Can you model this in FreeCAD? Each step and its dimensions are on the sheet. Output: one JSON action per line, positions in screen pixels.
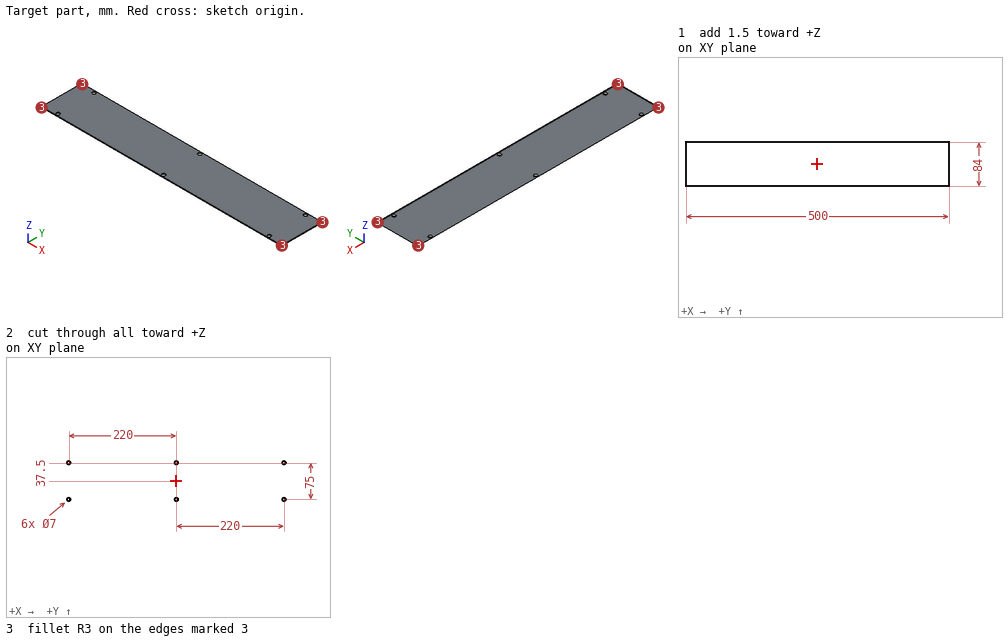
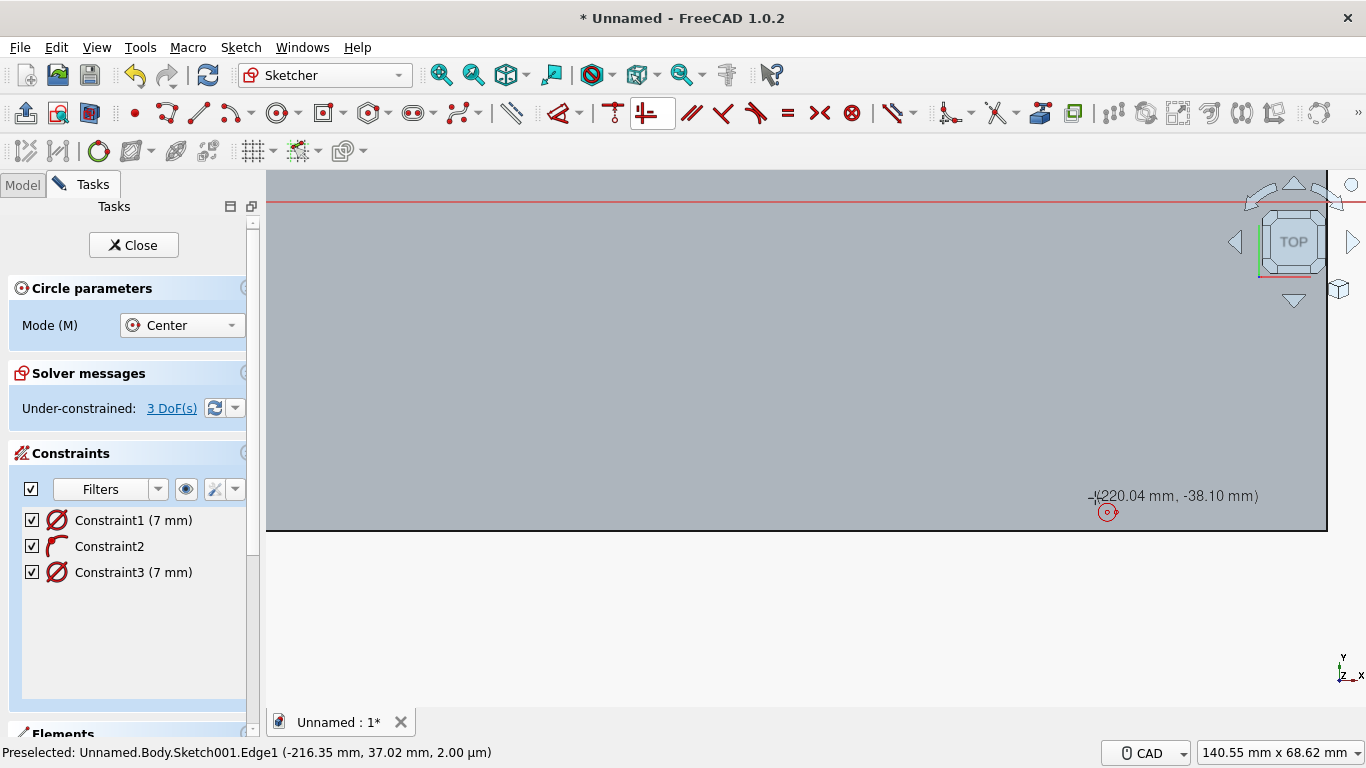
{"action": "scroll", "coordinate": [1096, 498], "scroll_direction": "down", "scroll_amount": 8}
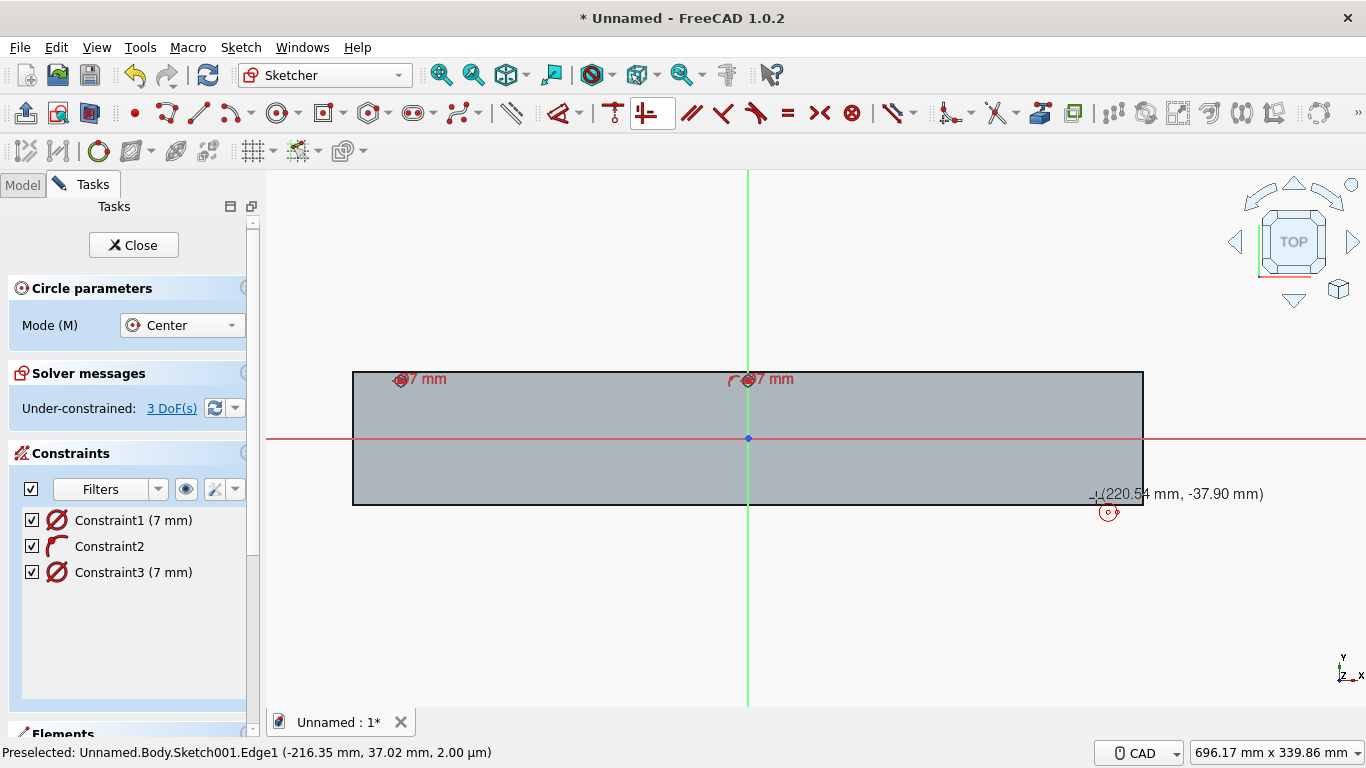
{"action": "left_click", "coordinate": [1096, 498]}
{"action": "mouse_move", "coordinate": [1100, 494]}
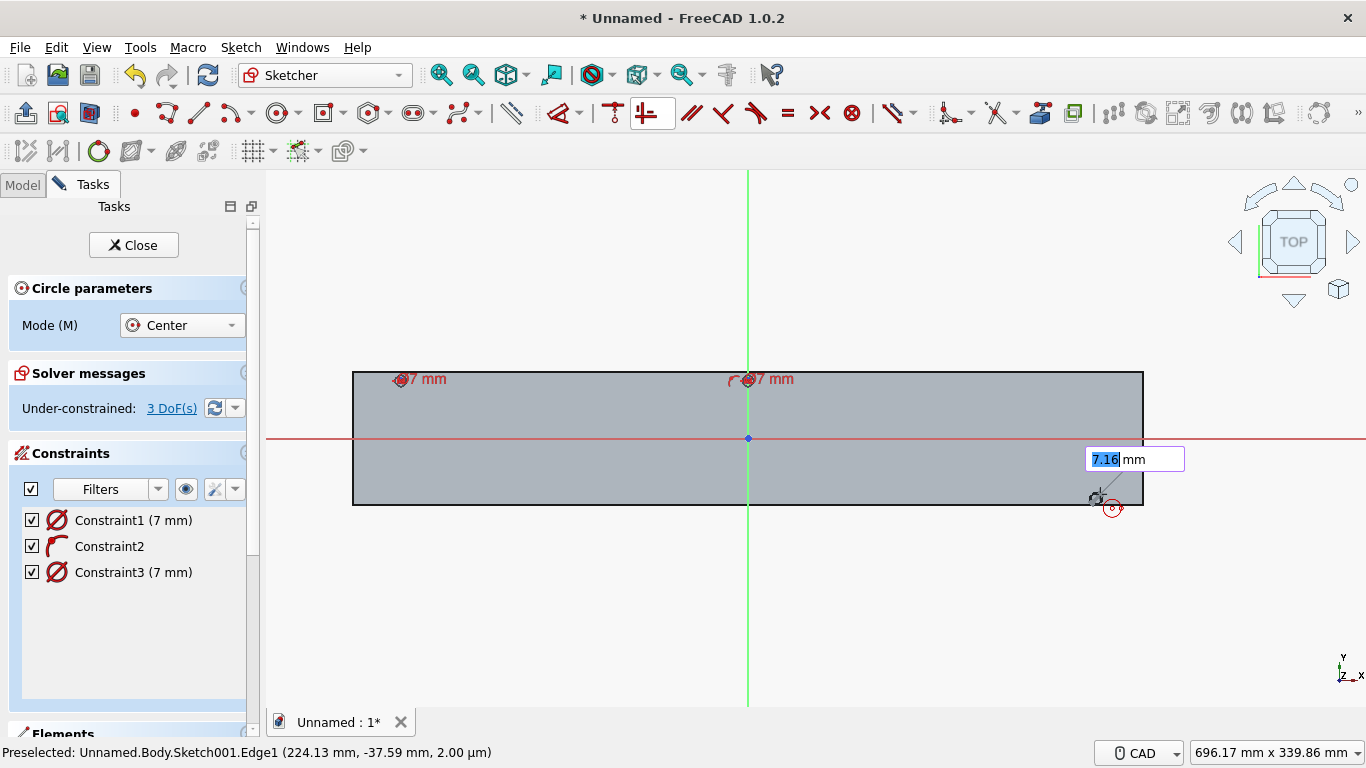
{"action": "type", "text": "7"}
{"action": "key", "text": "Return"}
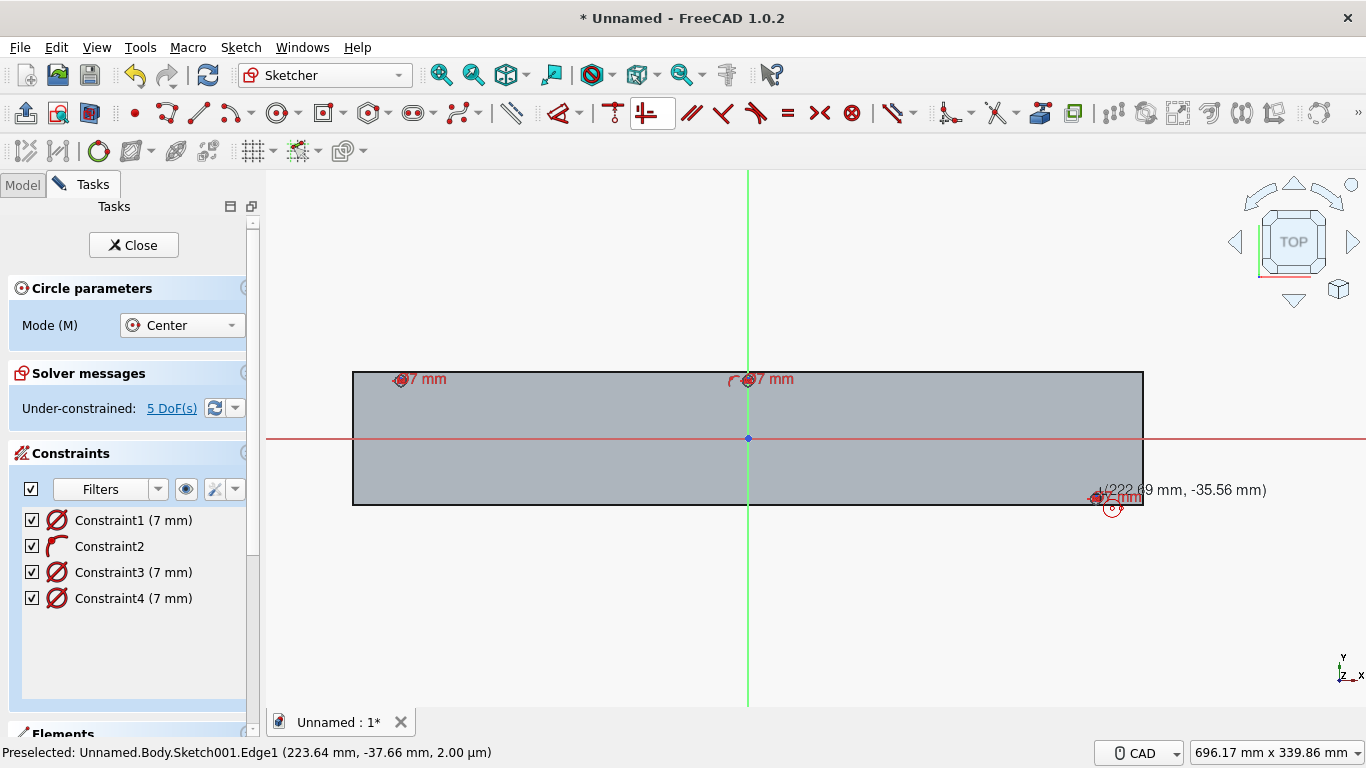
{"action": "scroll", "coordinate": [401, 498], "scroll_direction": "up", "scroll_amount": 8}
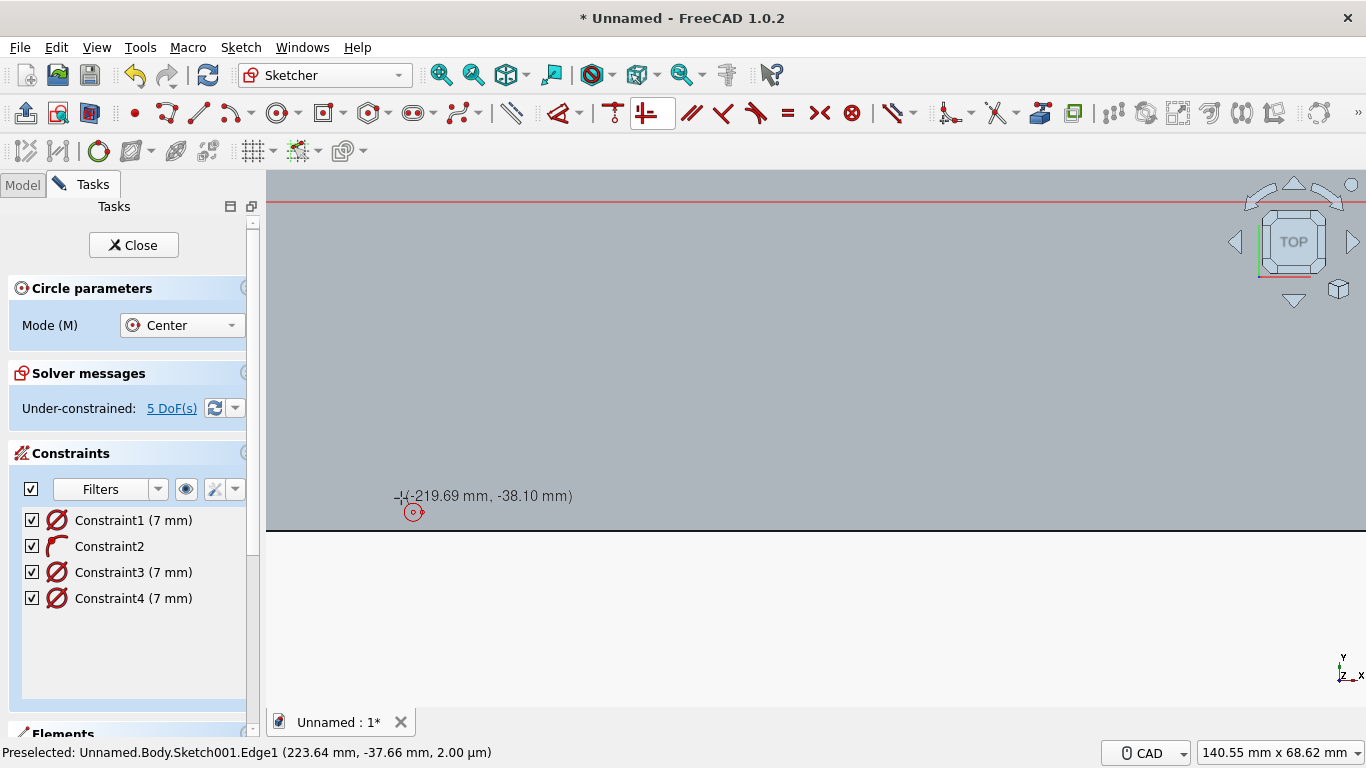
{"action": "scroll", "coordinate": [400, 498], "scroll_direction": "down", "scroll_amount": 8}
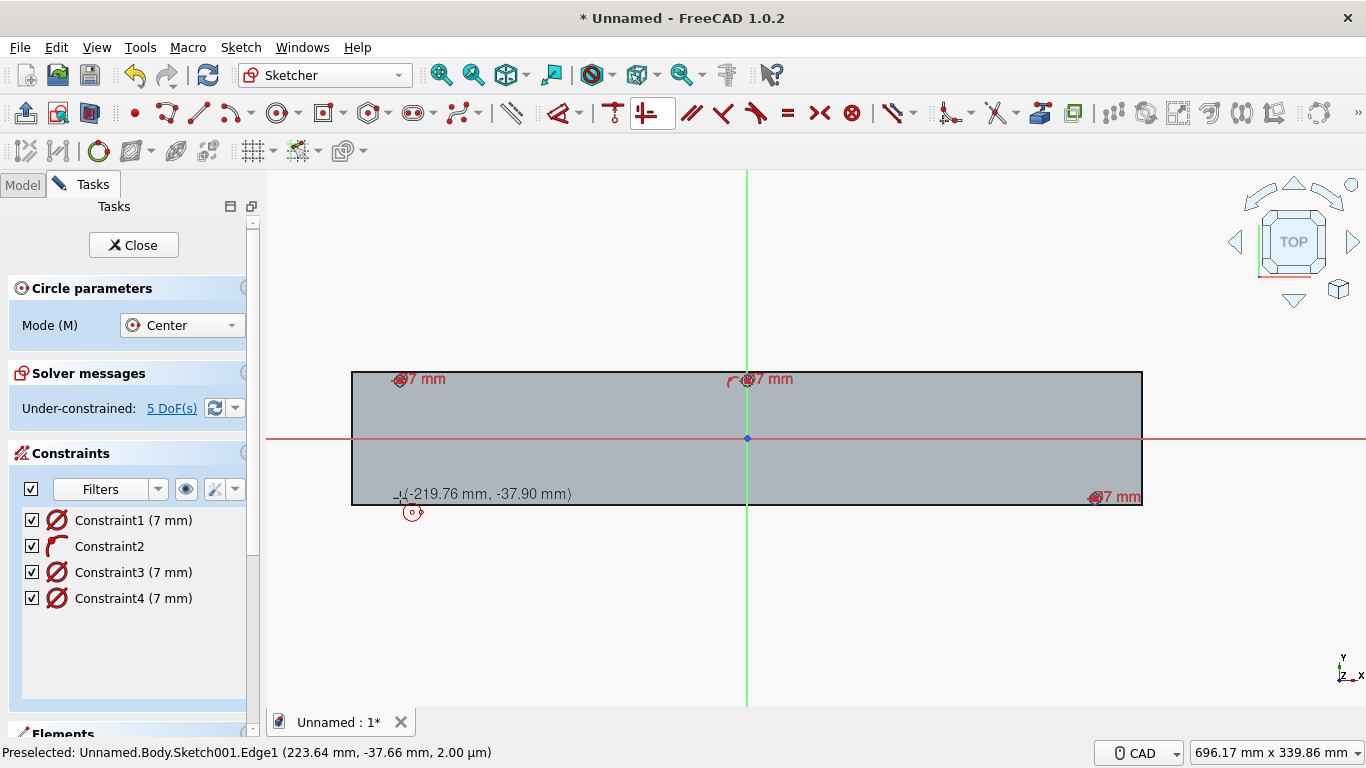
{"action": "left_click", "coordinate": [400, 498]}
{"action": "mouse_move", "coordinate": [404, 494]}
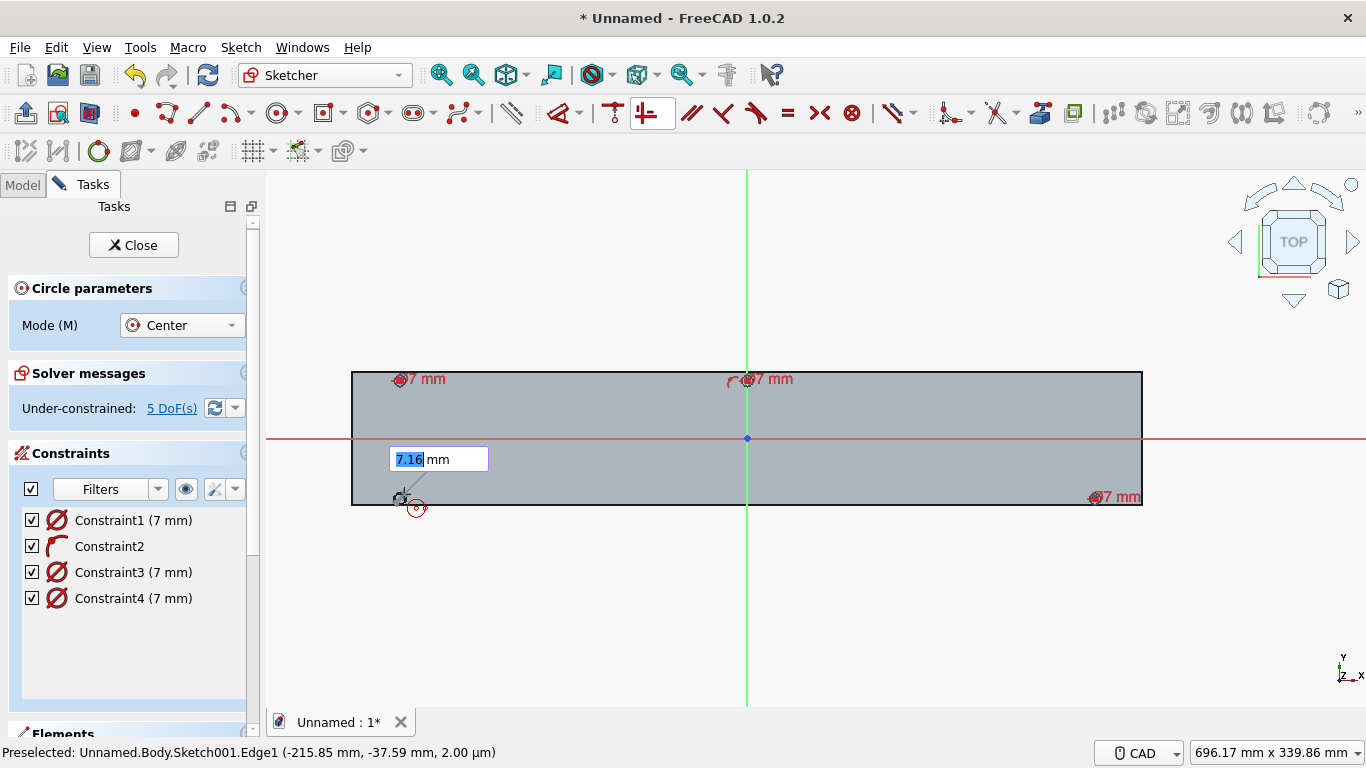
{"action": "type", "text": "7"}
{"action": "key", "text": "Return"}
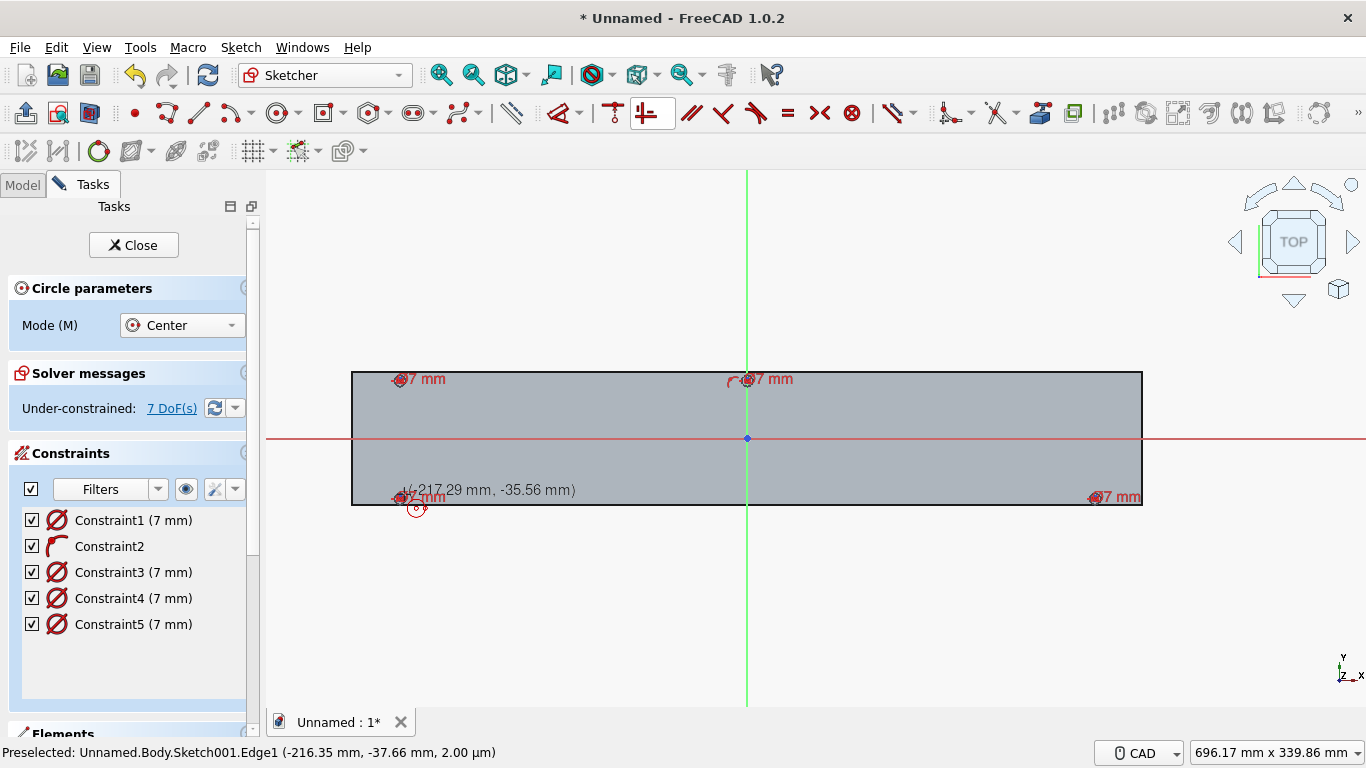
{"action": "scroll", "coordinate": [747, 498], "scroll_direction": "up", "scroll_amount": 8}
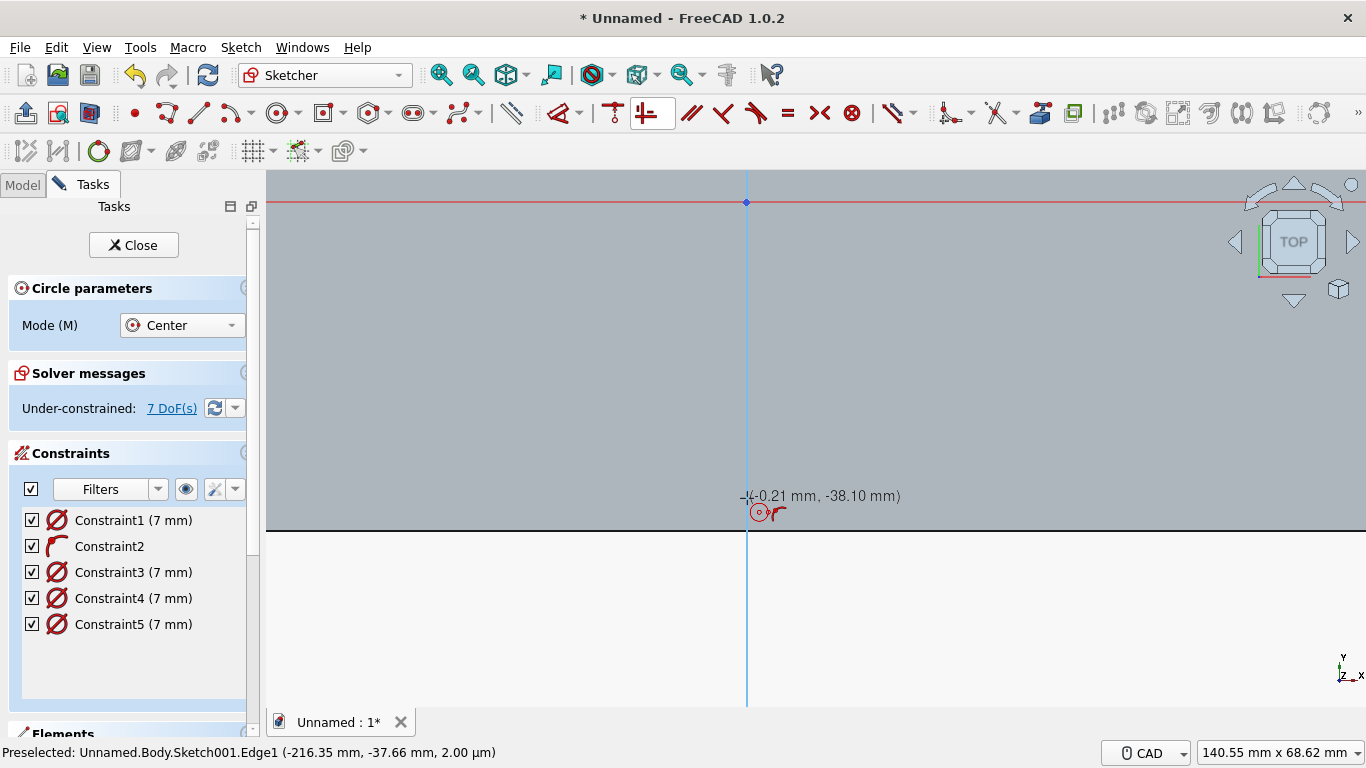
{"action": "scroll", "coordinate": [748, 498], "scroll_direction": "down", "scroll_amount": 8}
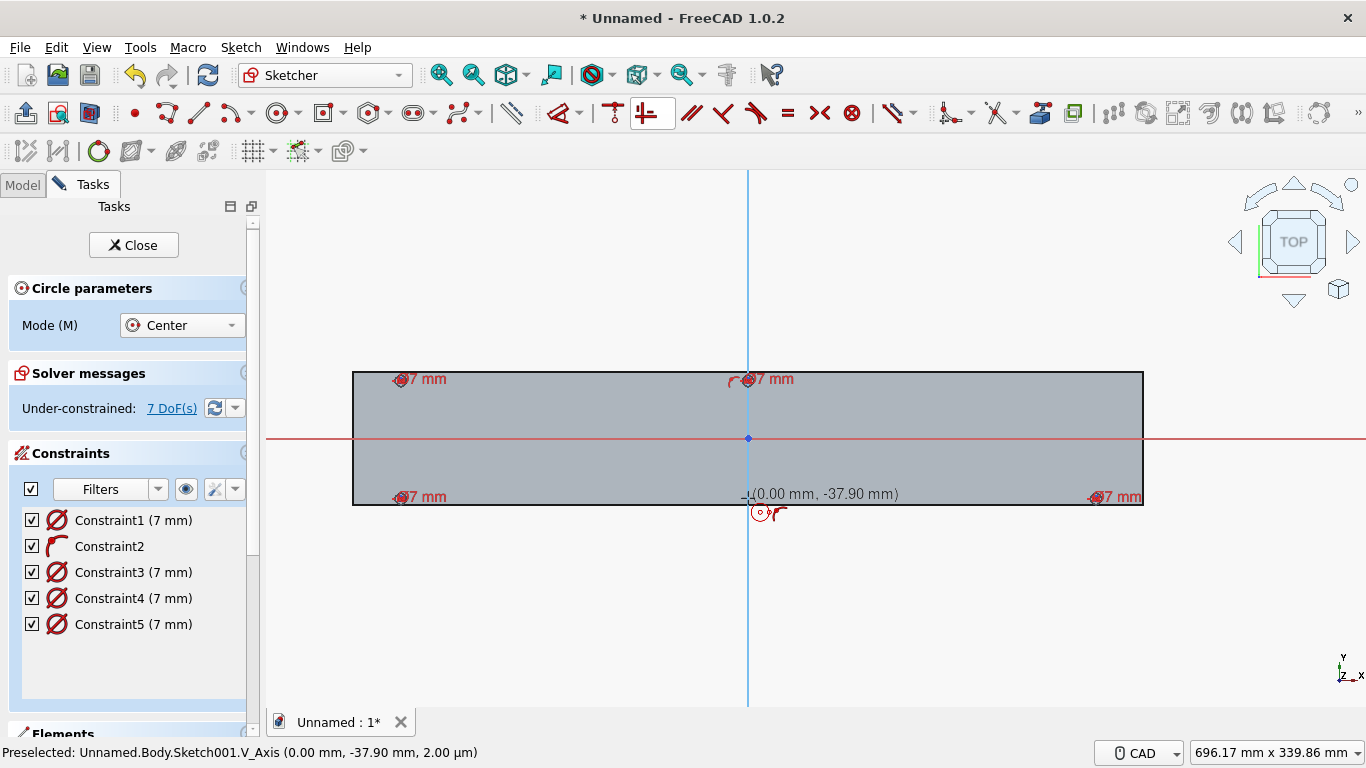
{"action": "left_click", "coordinate": [748, 498]}